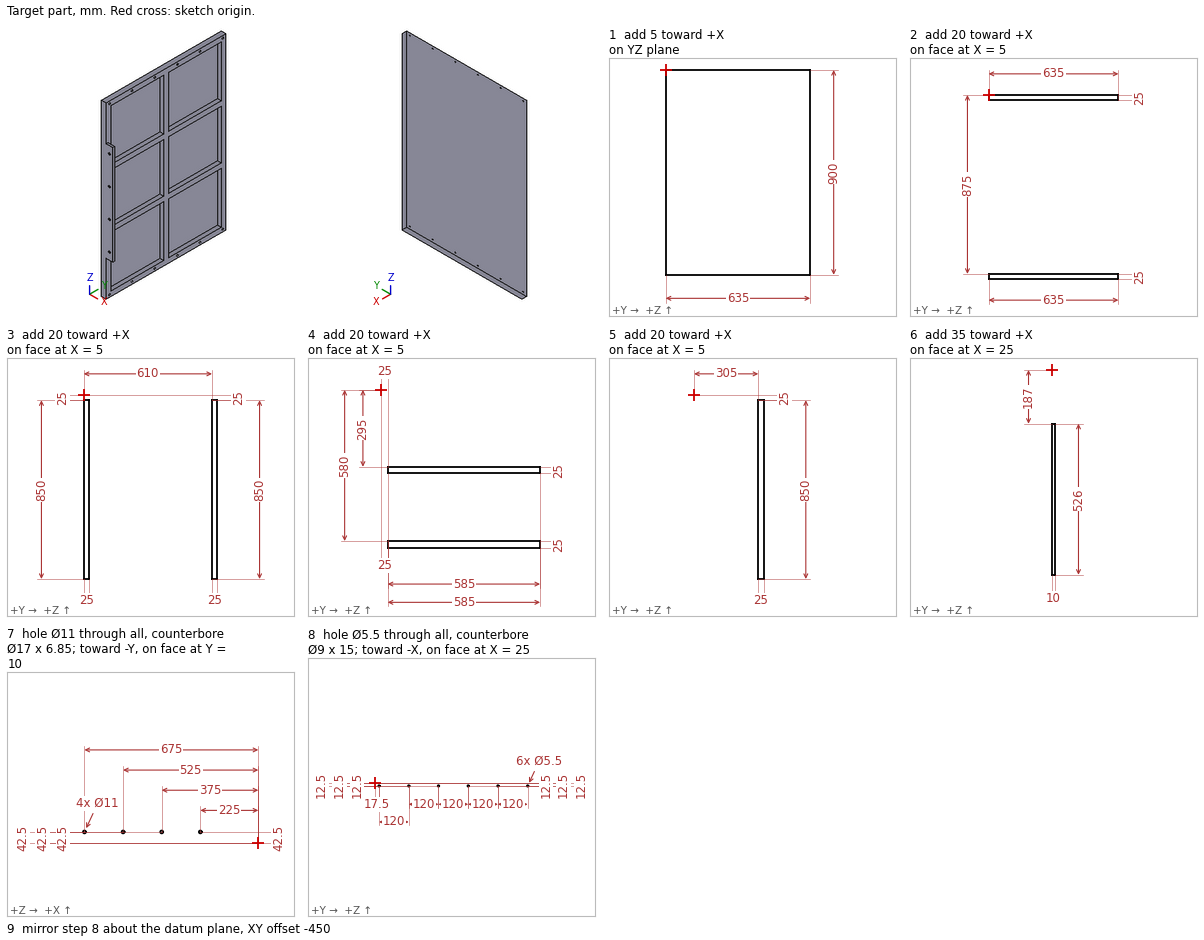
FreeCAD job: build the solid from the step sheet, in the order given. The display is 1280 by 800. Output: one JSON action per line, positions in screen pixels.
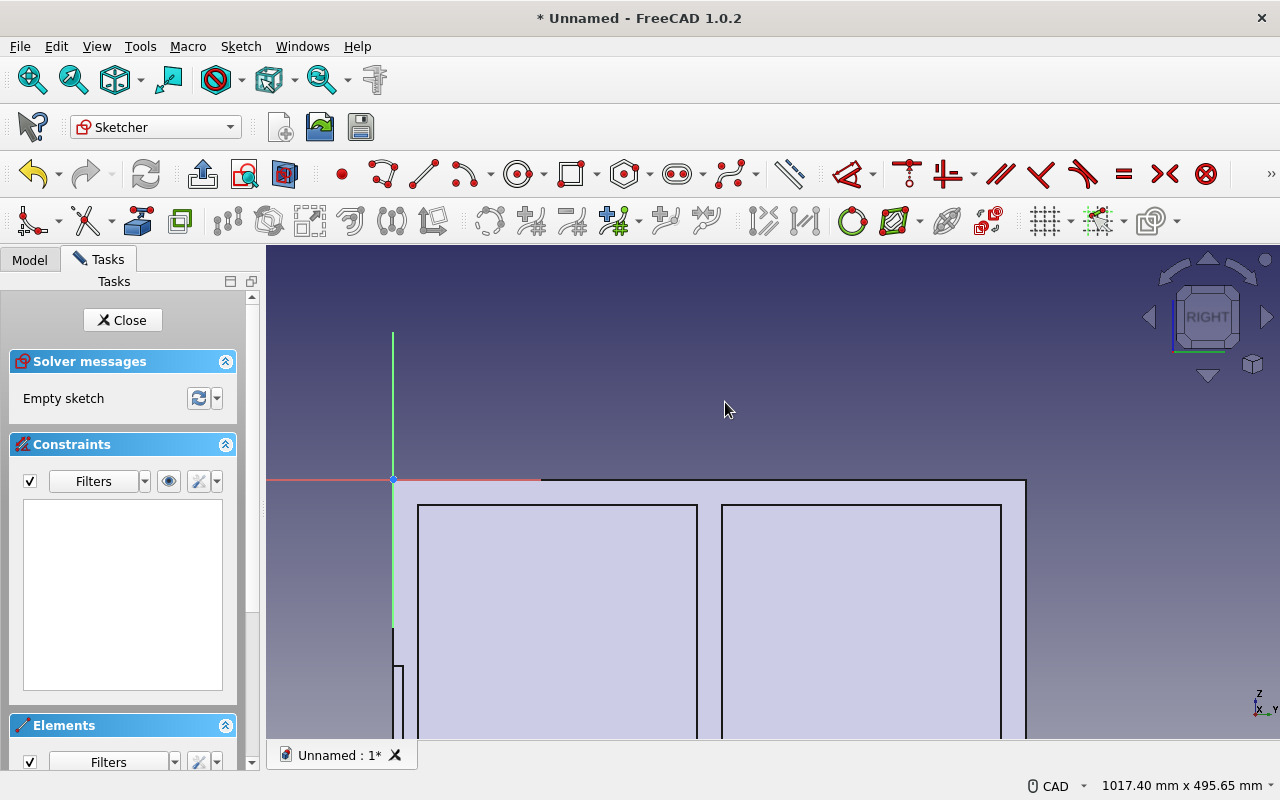
{"action": "left_click", "coordinate": [518, 174]}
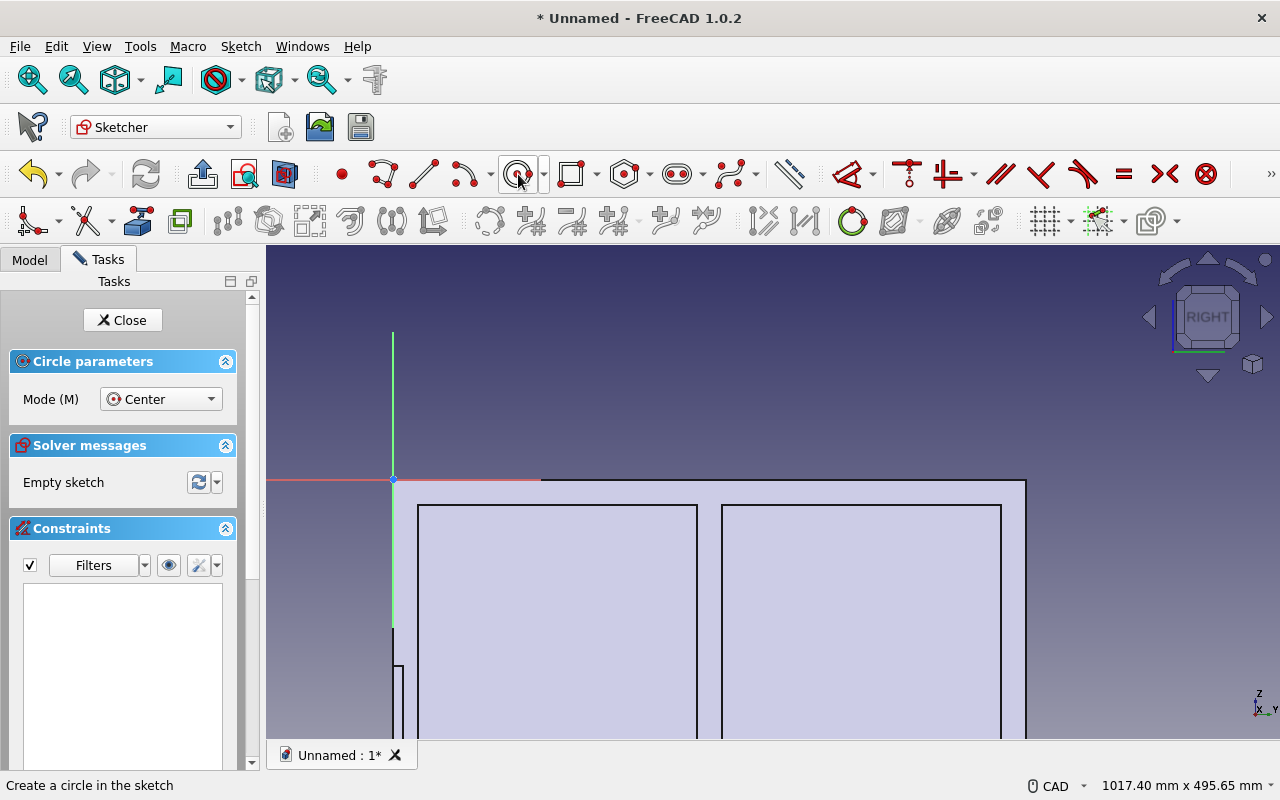
{"action": "scroll", "coordinate": [1009, 492], "scroll_direction": "up", "scroll_amount": 11}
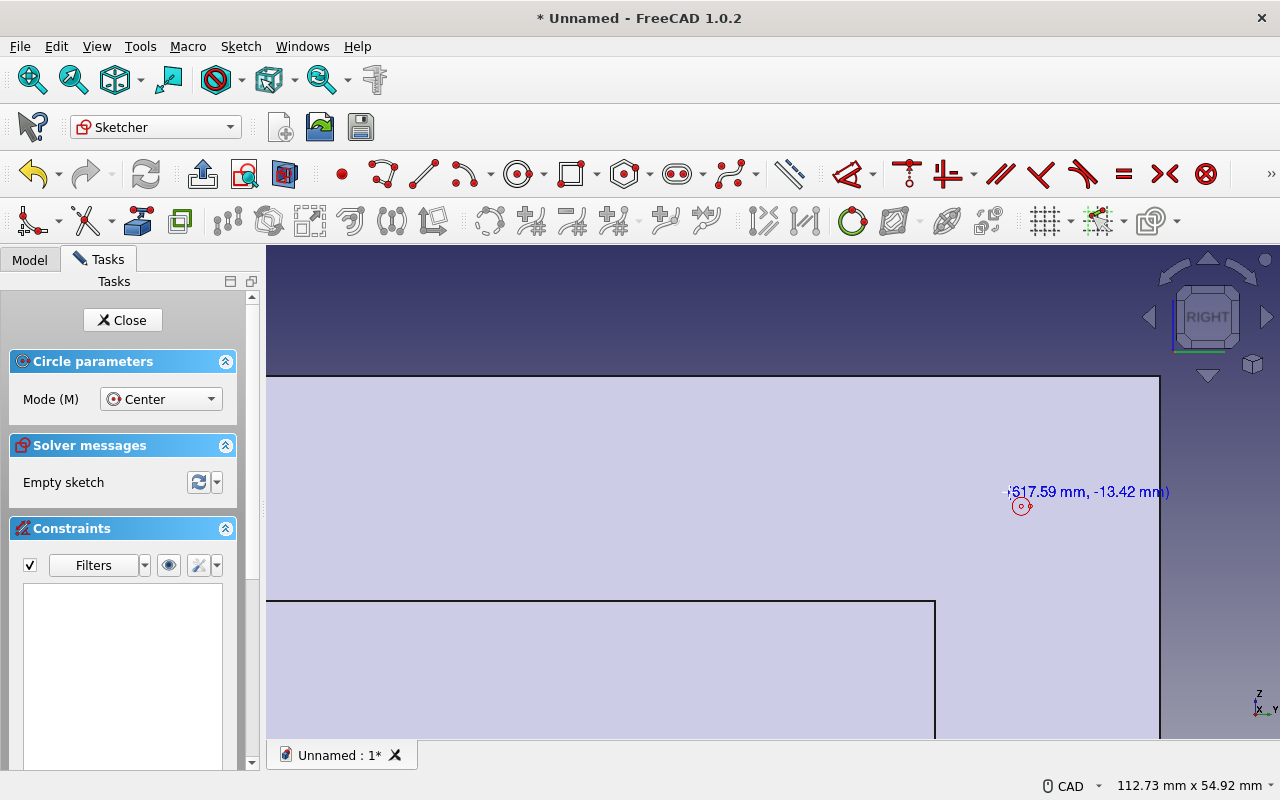
{"action": "scroll", "coordinate": [1012, 498], "scroll_direction": "down", "scroll_amount": 11}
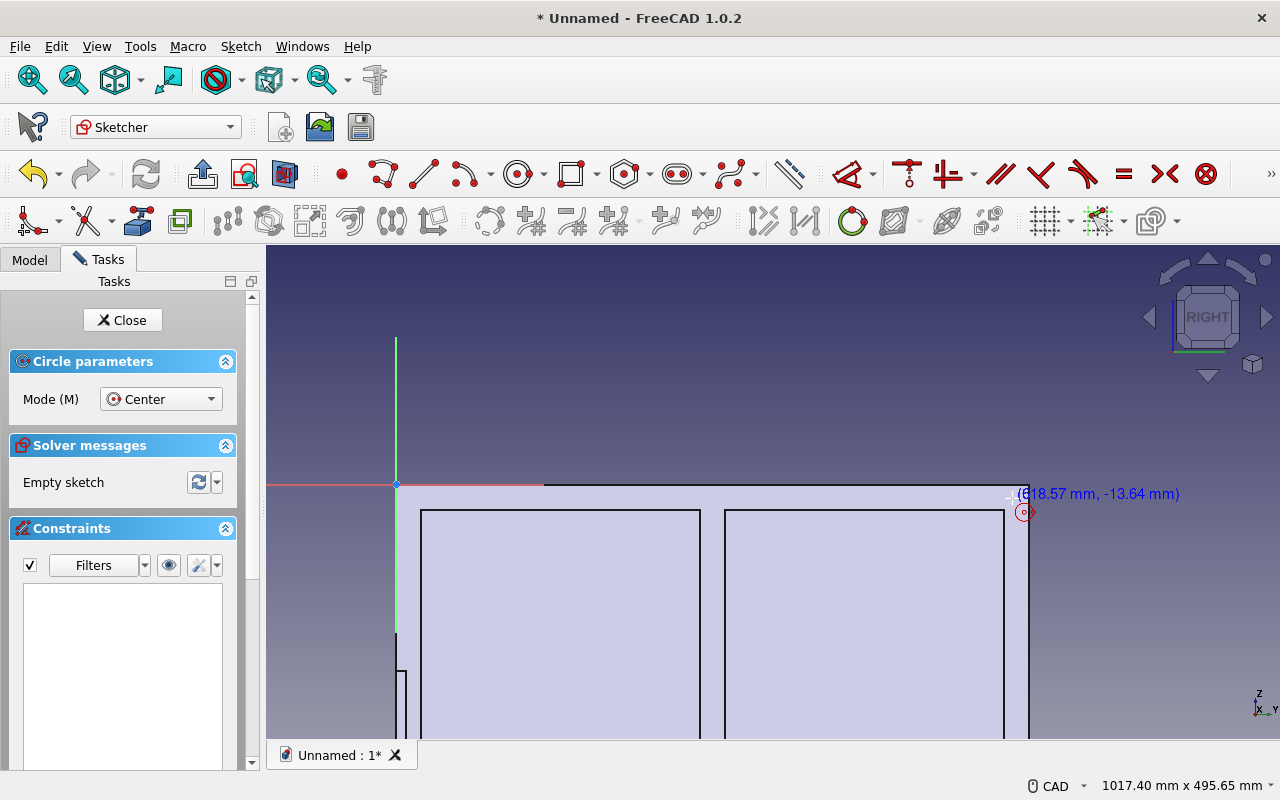
{"action": "scroll", "coordinate": [1012, 497], "scroll_direction": "up", "scroll_amount": 2}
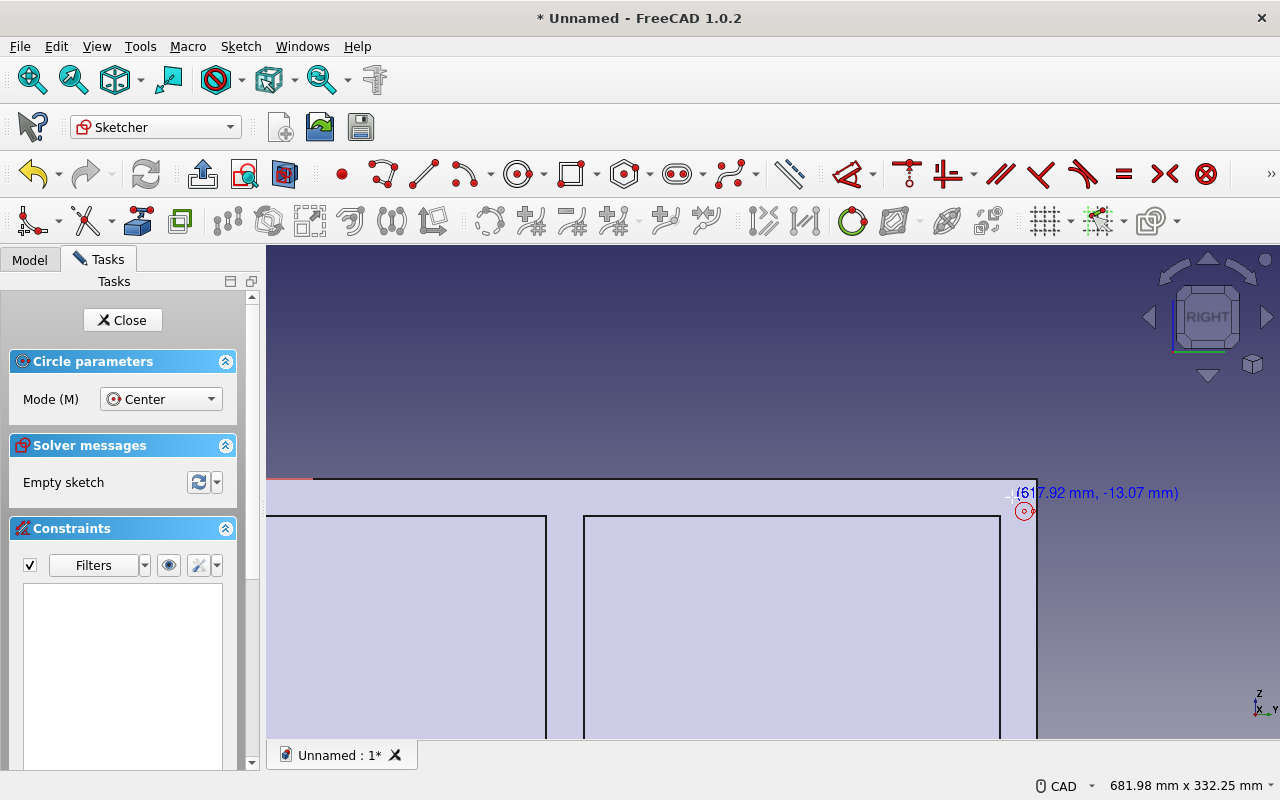
{"action": "left_click", "coordinate": [1011, 497]}
{"action": "mouse_move", "coordinate": [1014, 494]}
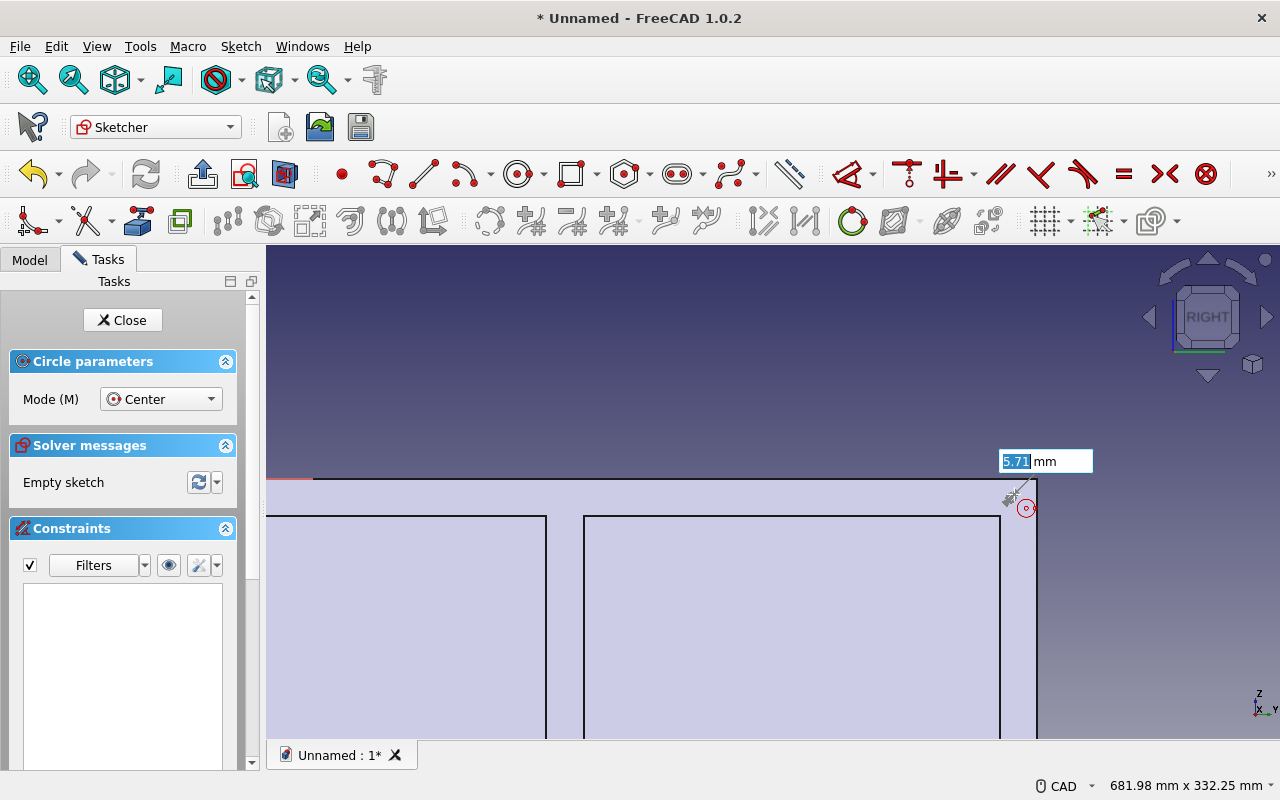
{"action": "type", "text": "5.5"}
{"action": "key", "text": "Return"}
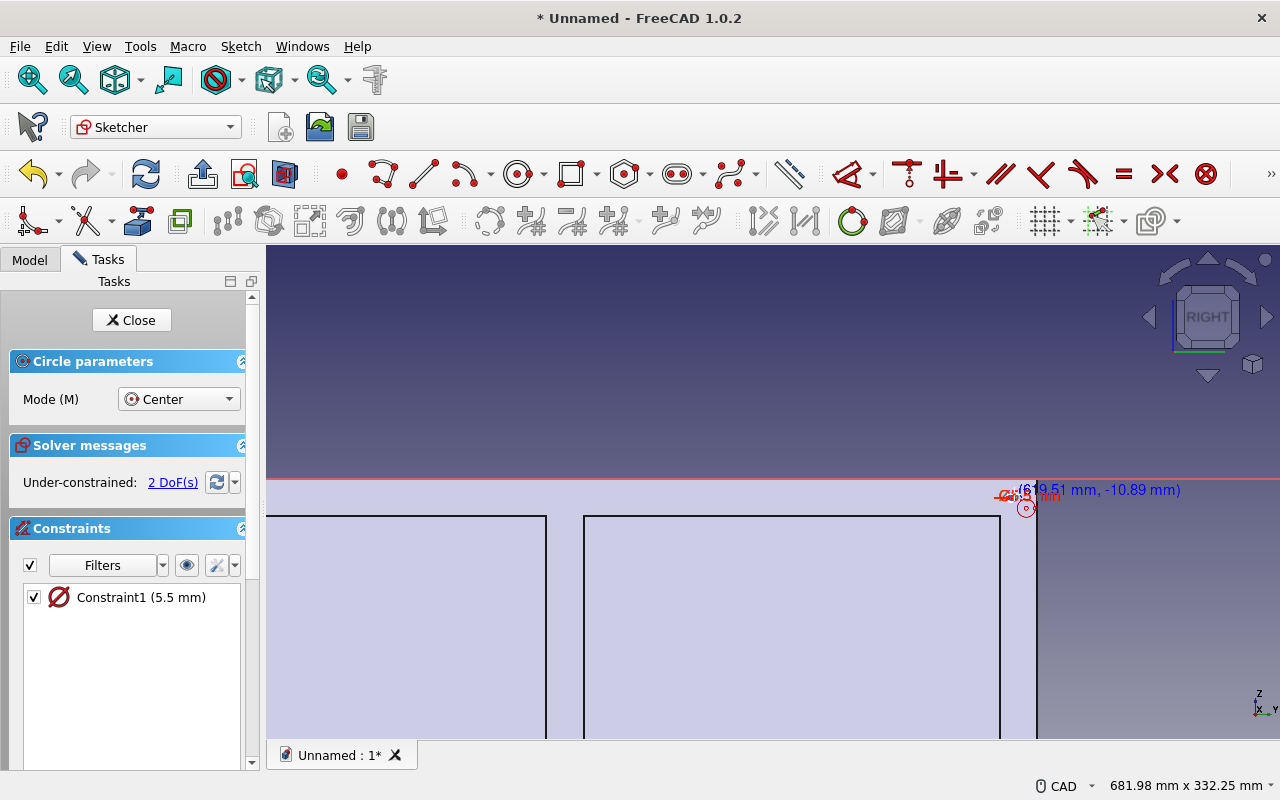
{"action": "scroll", "coordinate": [833, 497], "scroll_direction": "up", "scroll_amount": 9}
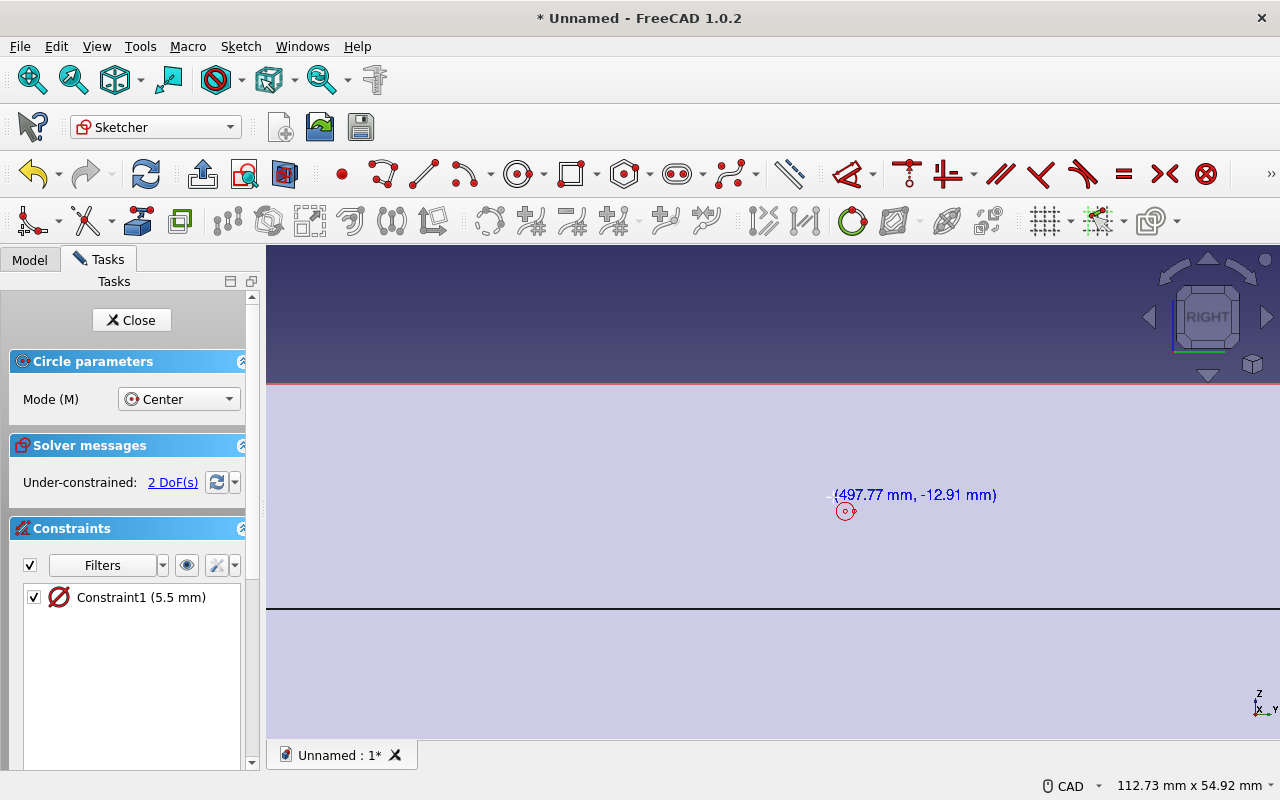
{"action": "scroll", "coordinate": [899, 497], "scroll_direction": "down", "scroll_amount": 11}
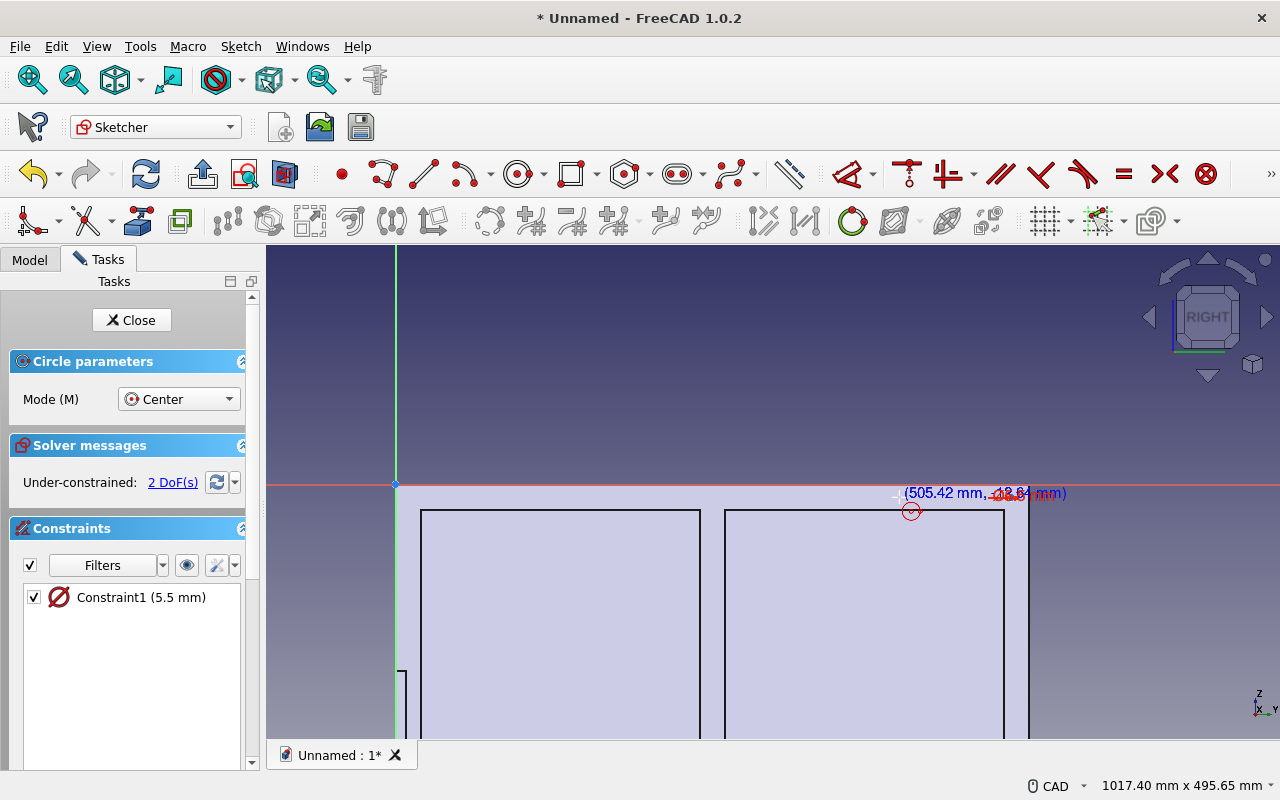
{"action": "scroll", "coordinate": [892, 497], "scroll_direction": "up", "scroll_amount": 2}